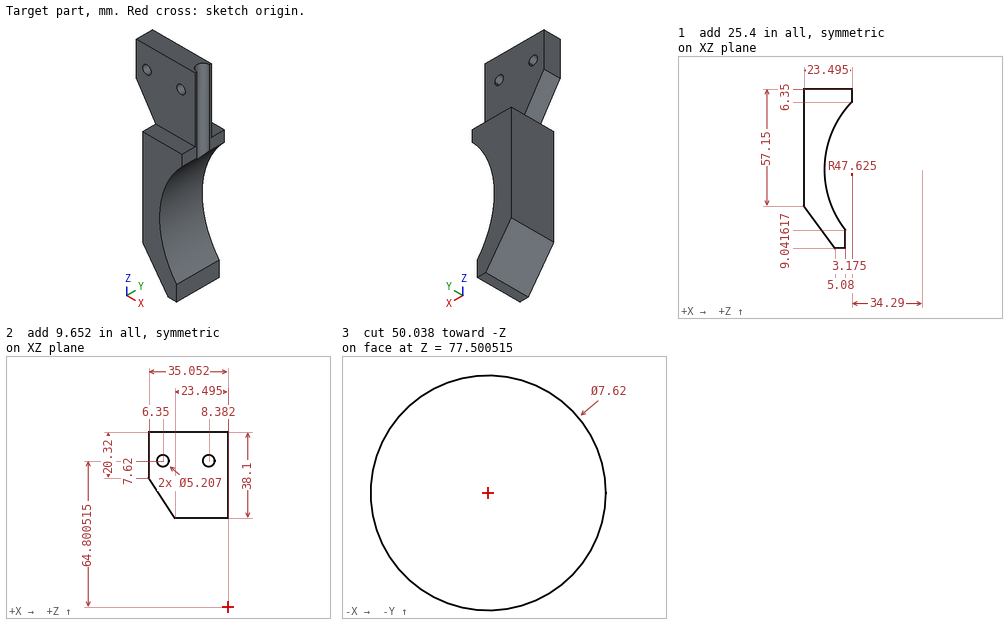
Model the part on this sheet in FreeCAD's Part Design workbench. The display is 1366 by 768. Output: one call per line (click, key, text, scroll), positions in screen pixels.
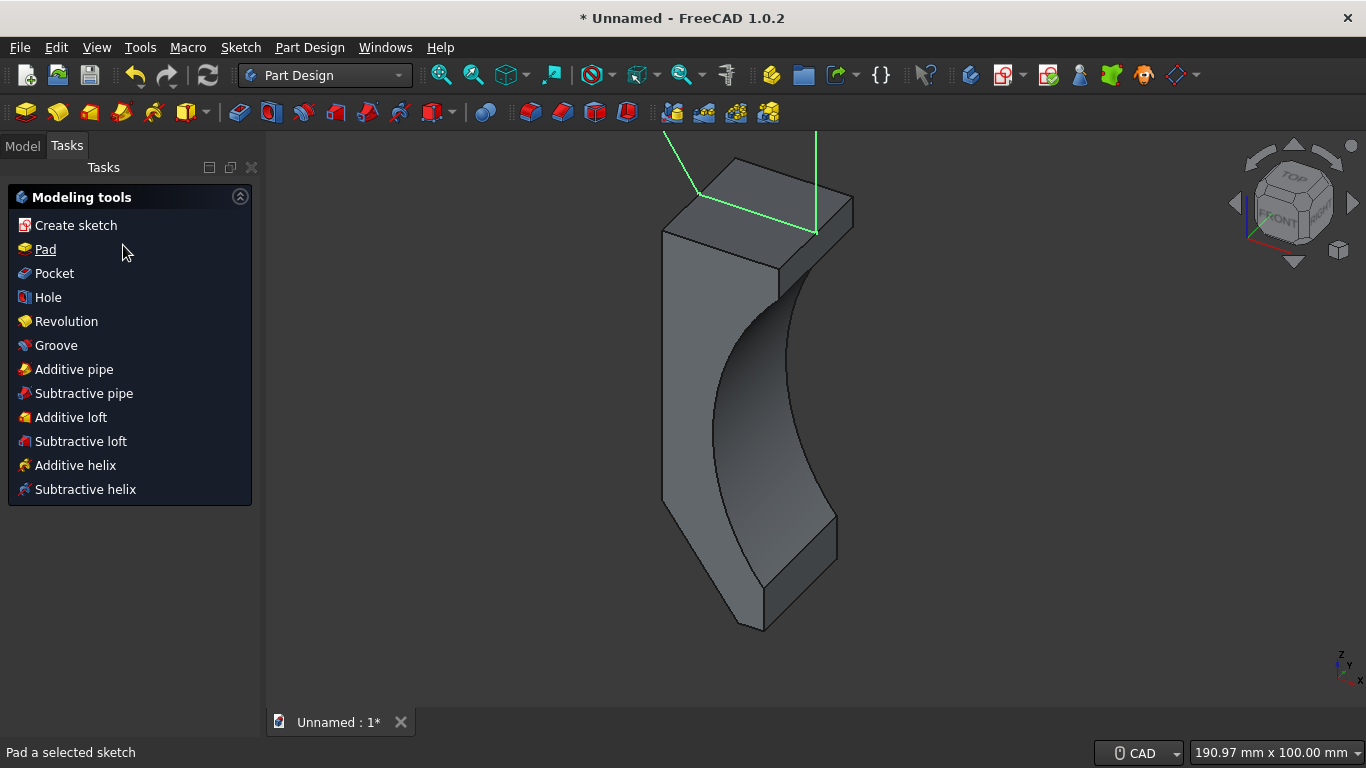
click(26, 112)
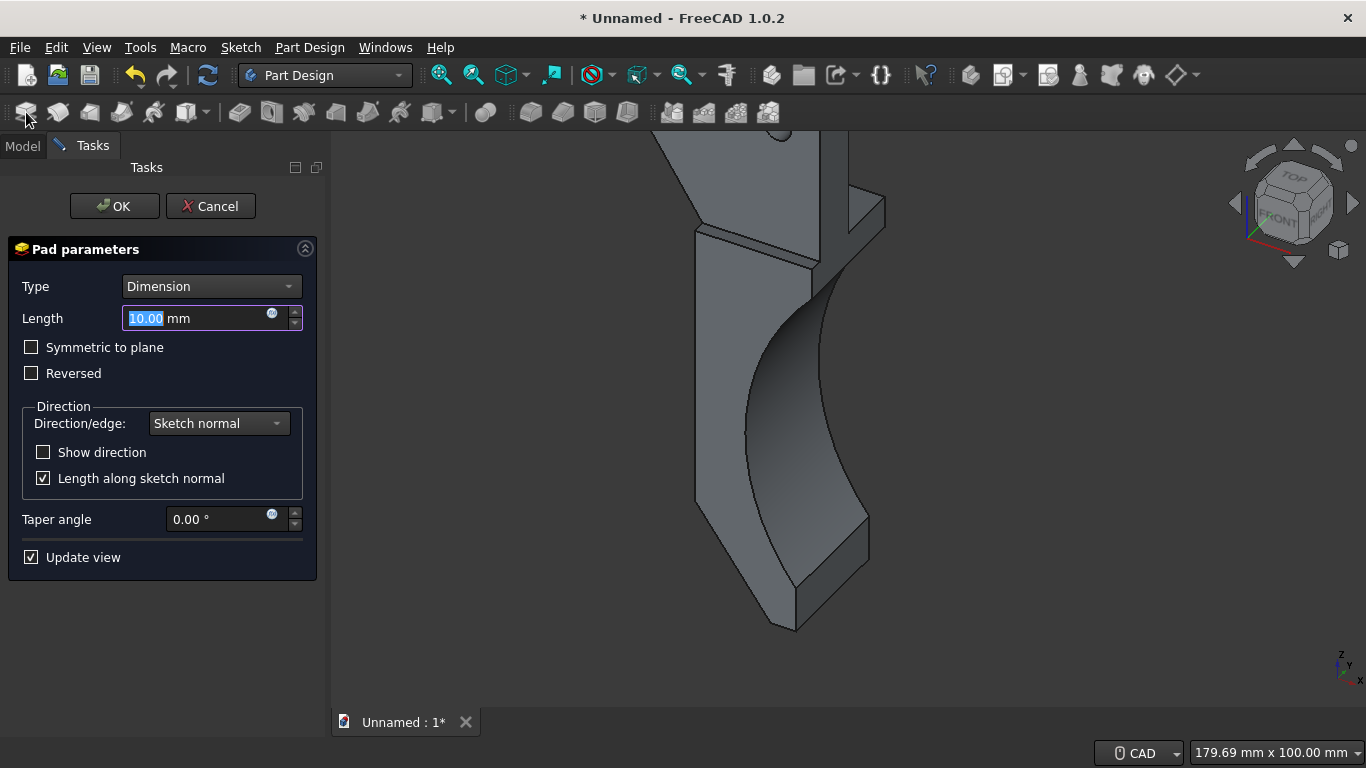
text(9.652)
key(Tab)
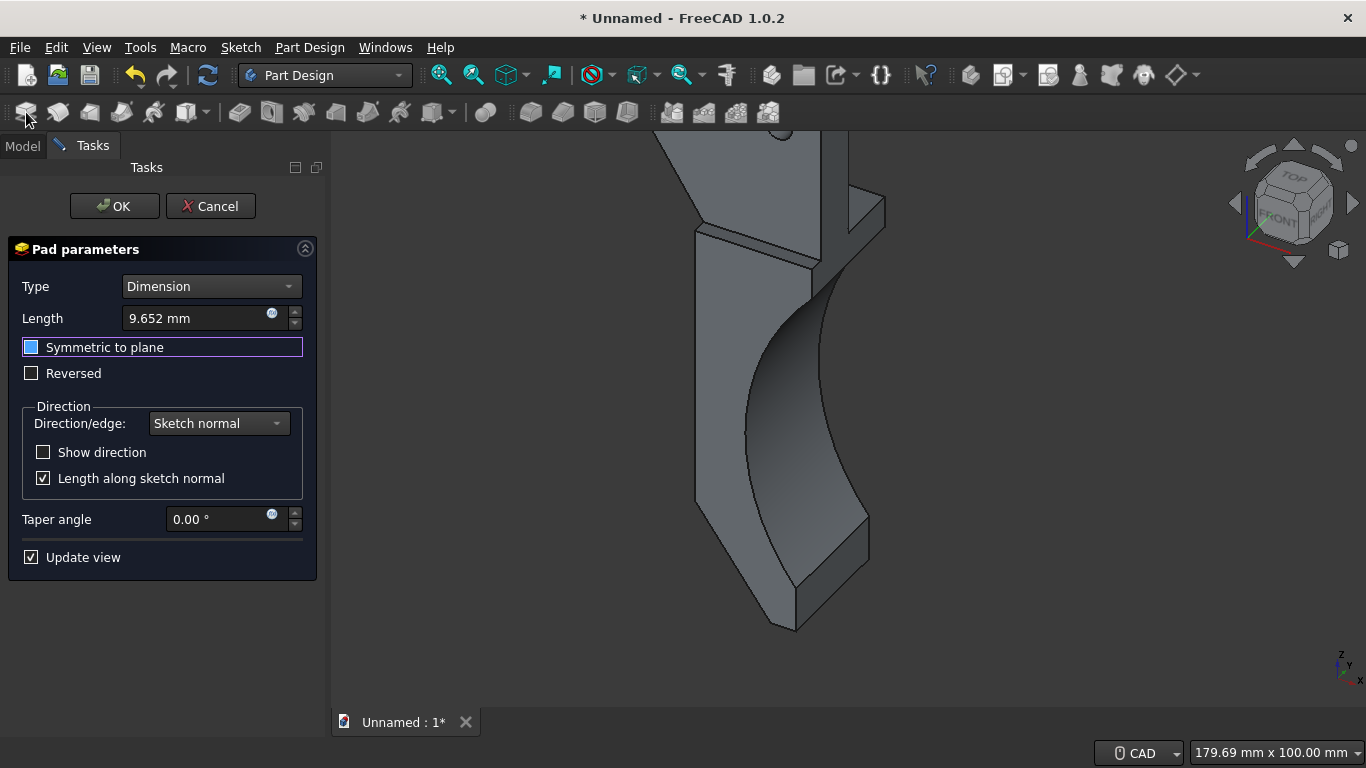
click(30, 347)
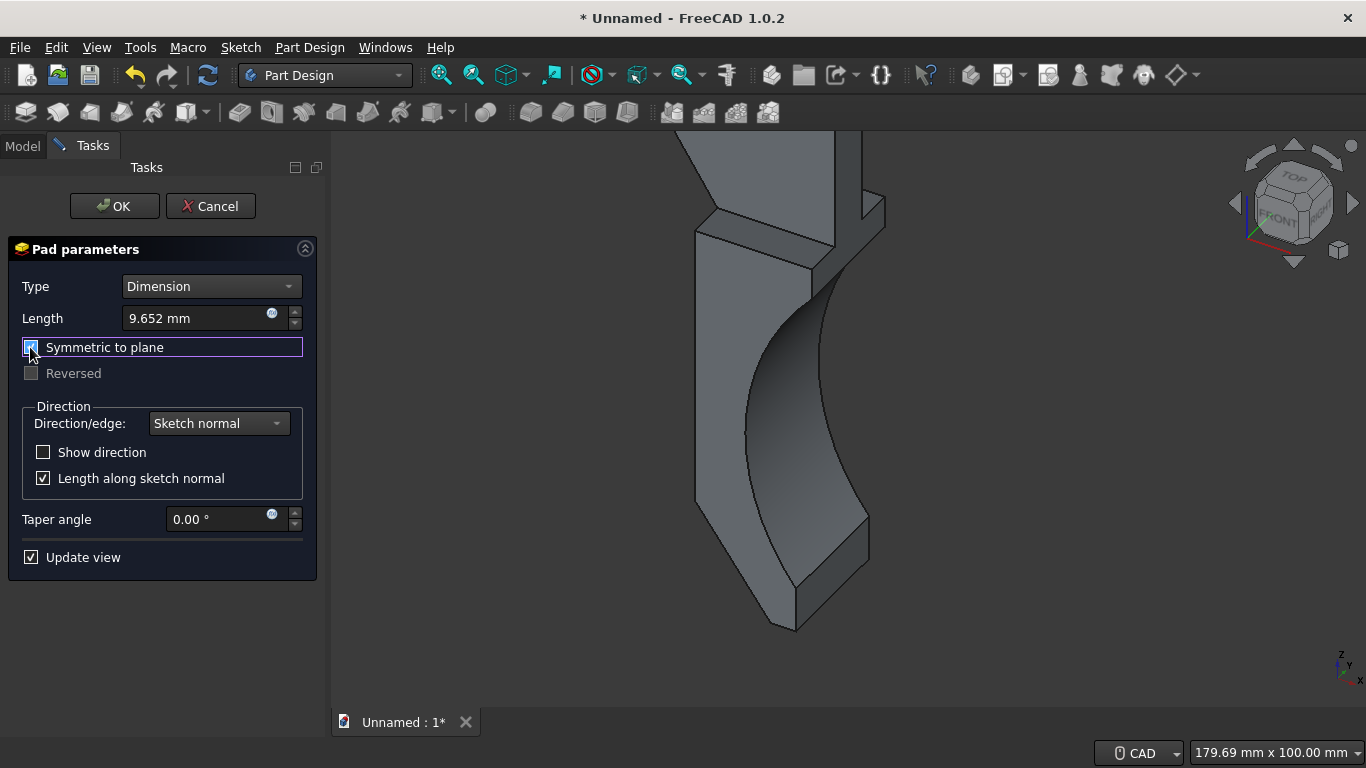
click(115, 206)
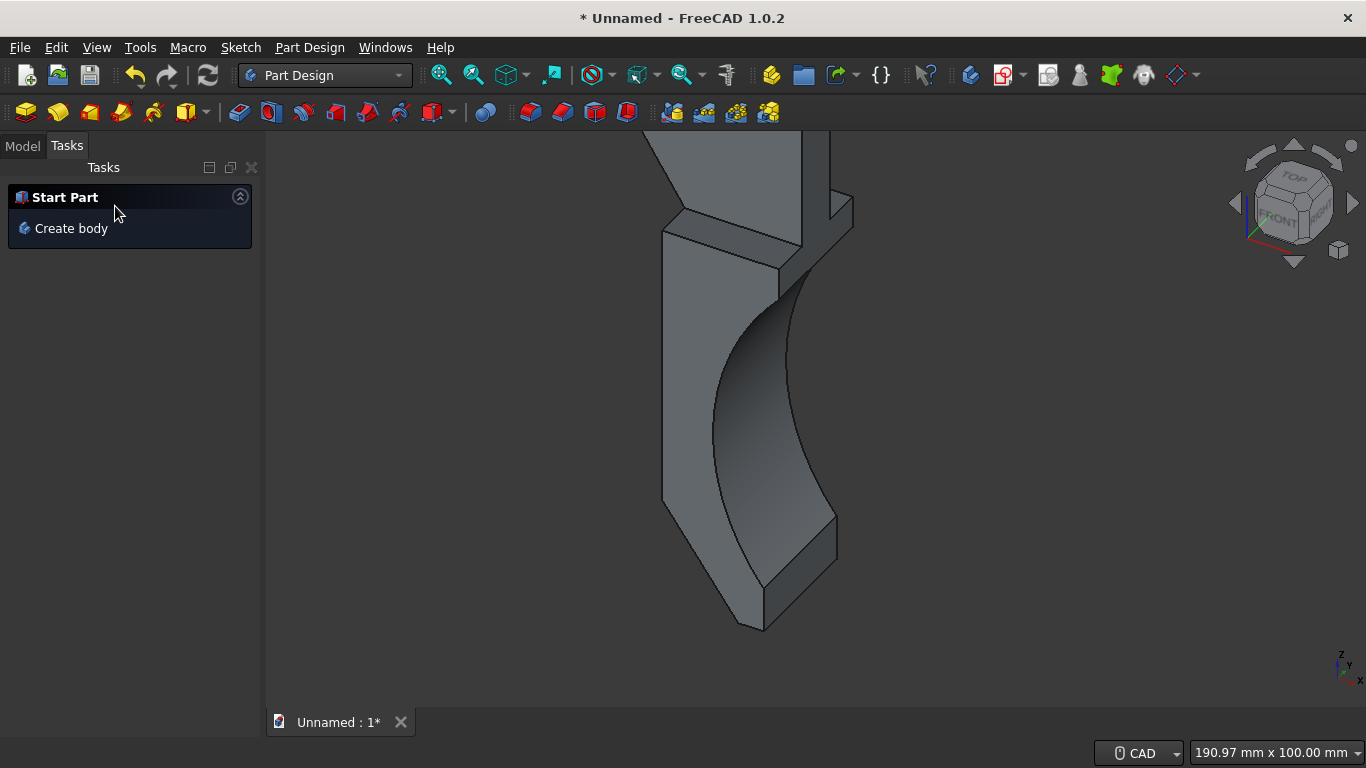
click(442, 76)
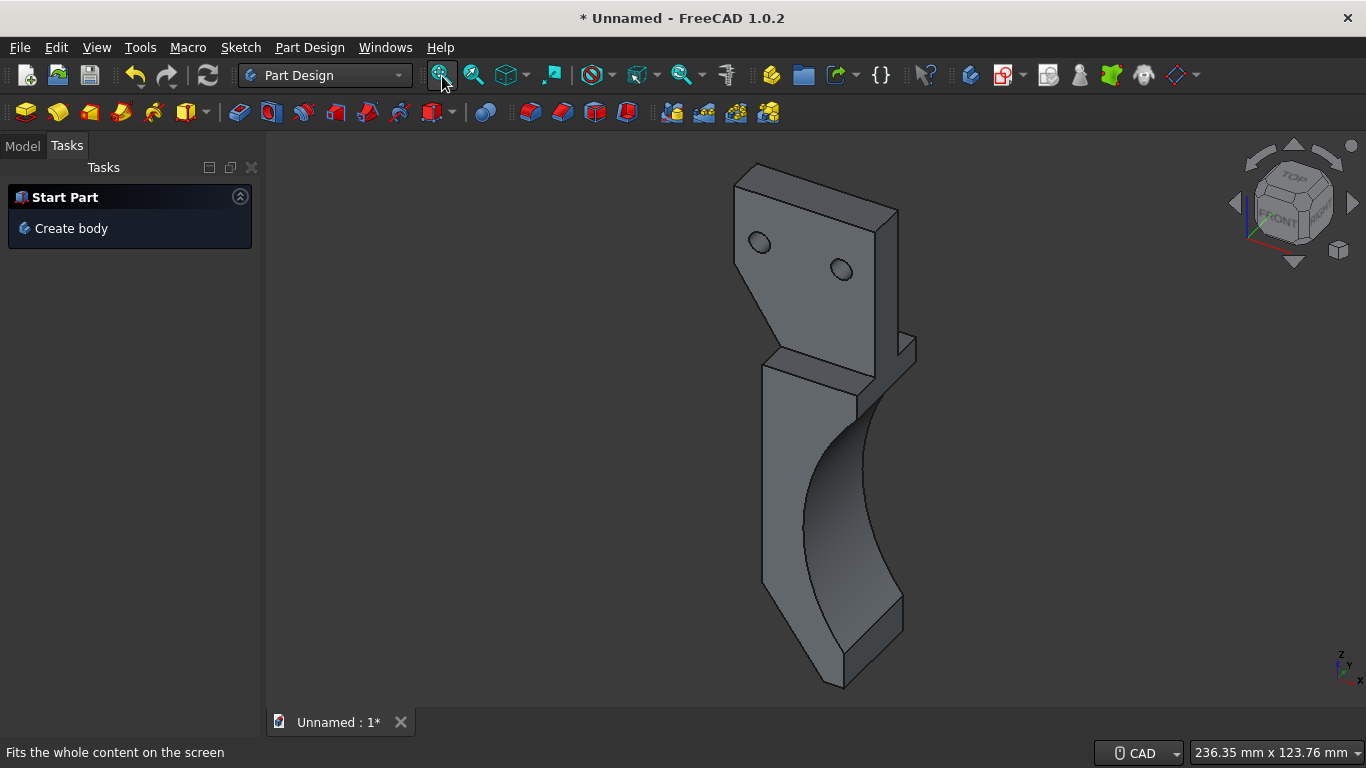
click(856, 210)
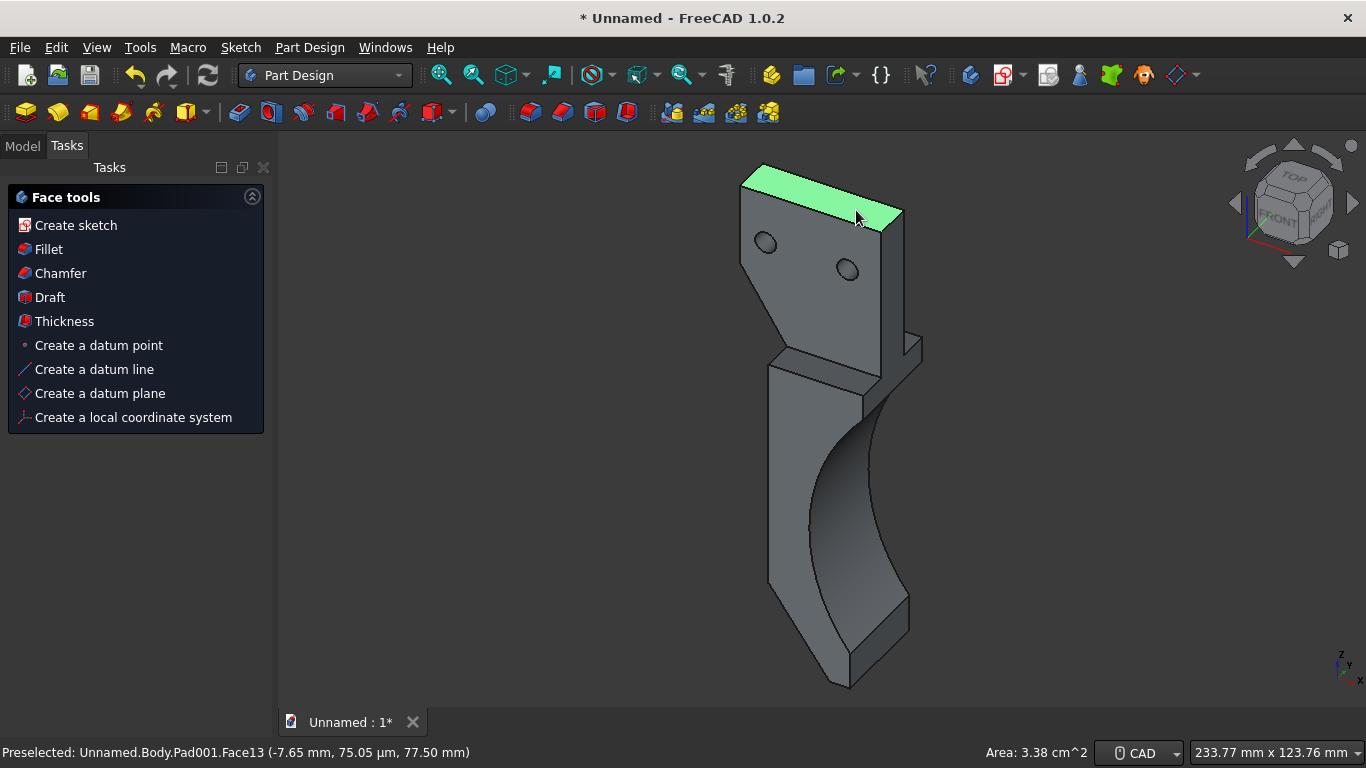
click(1004, 76)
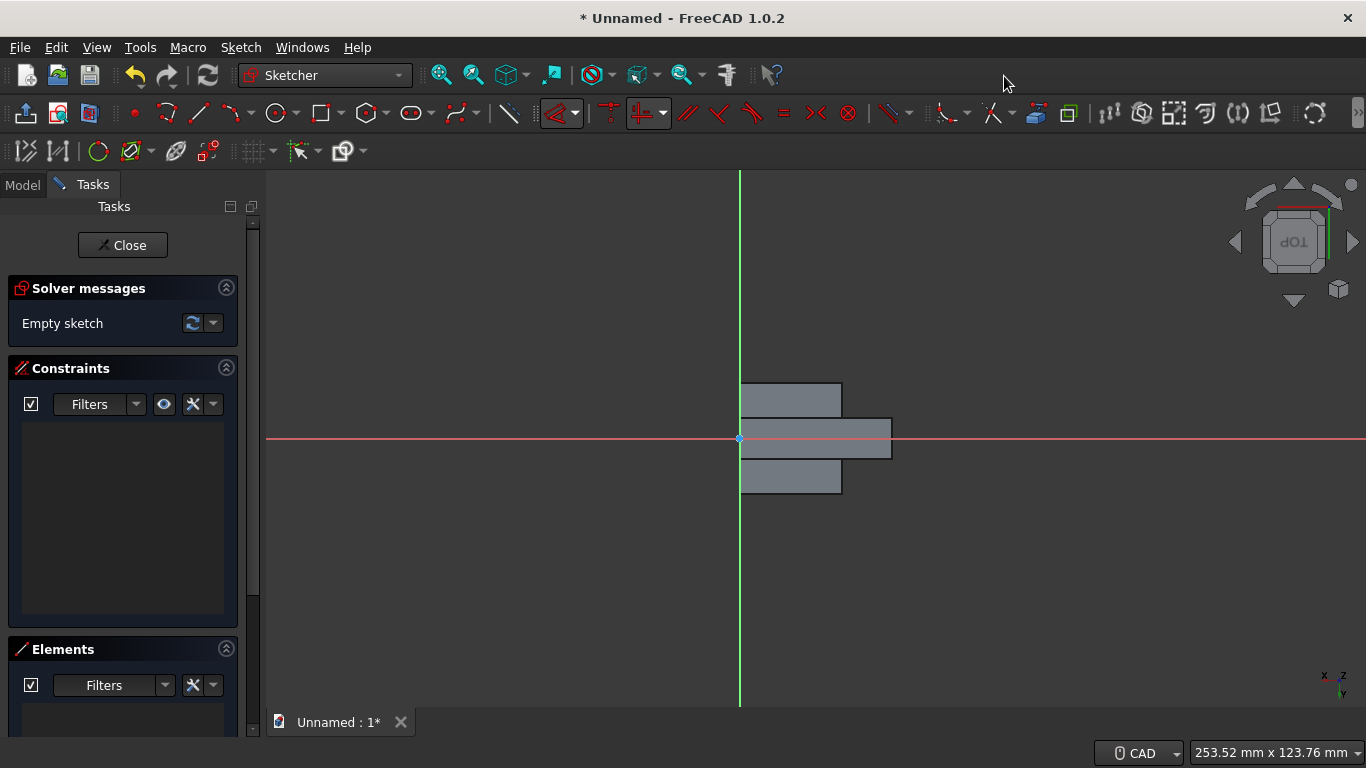
scroll(739, 439, up, 12)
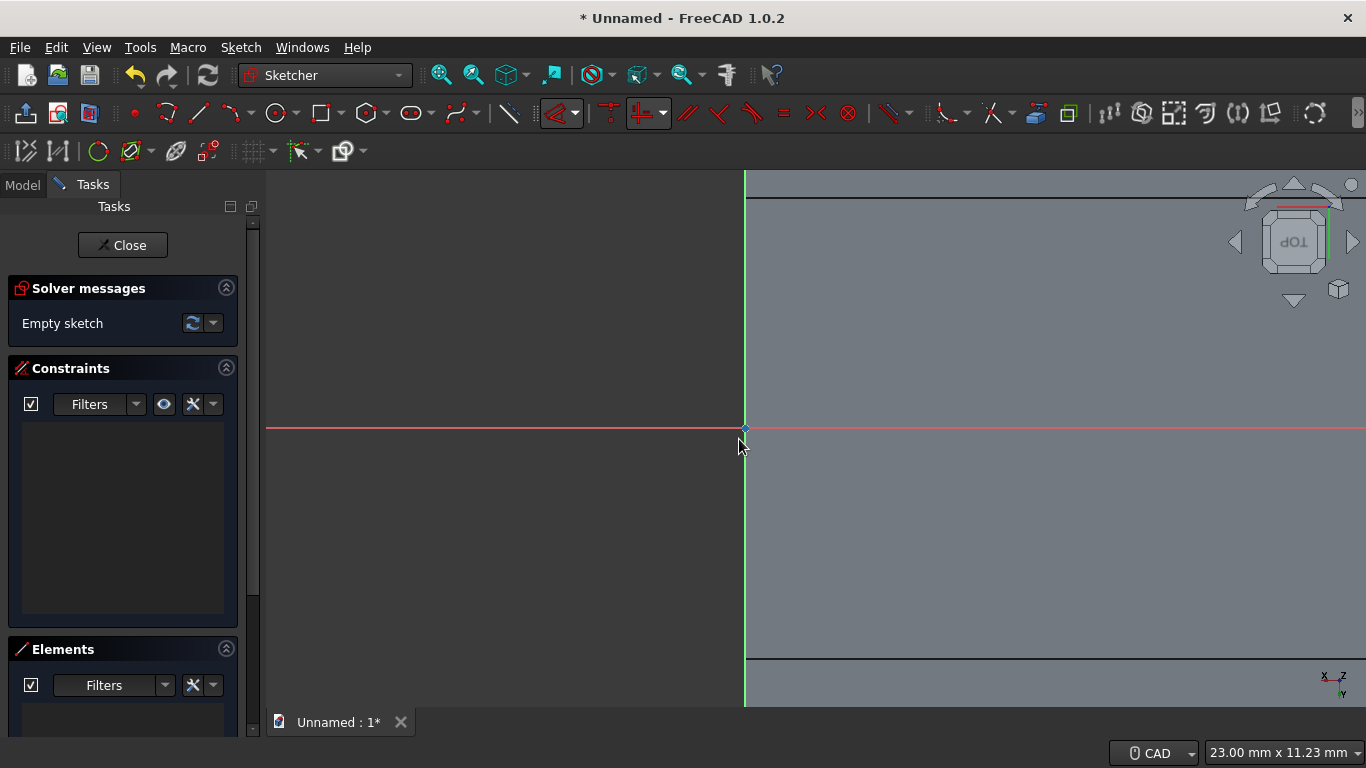
click(276, 114)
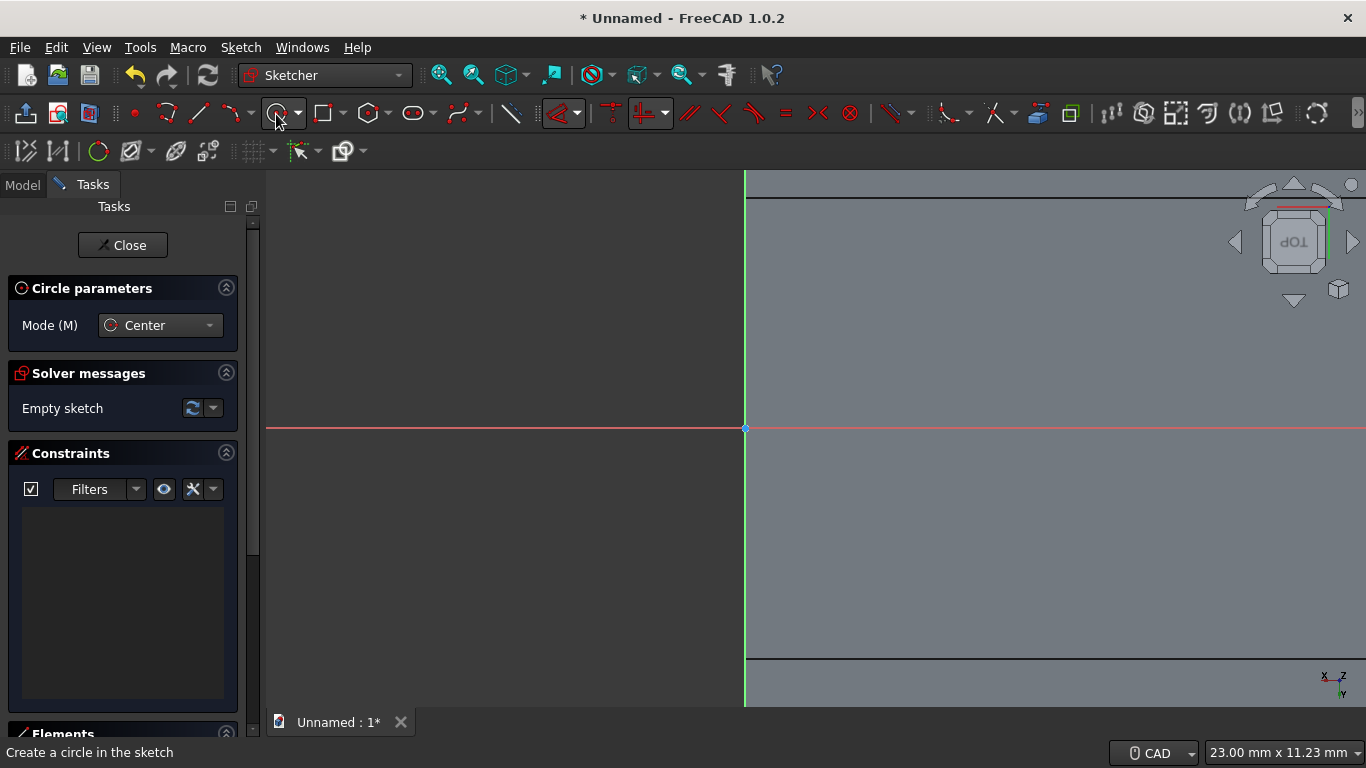
click(745, 428)
move(874, 300)